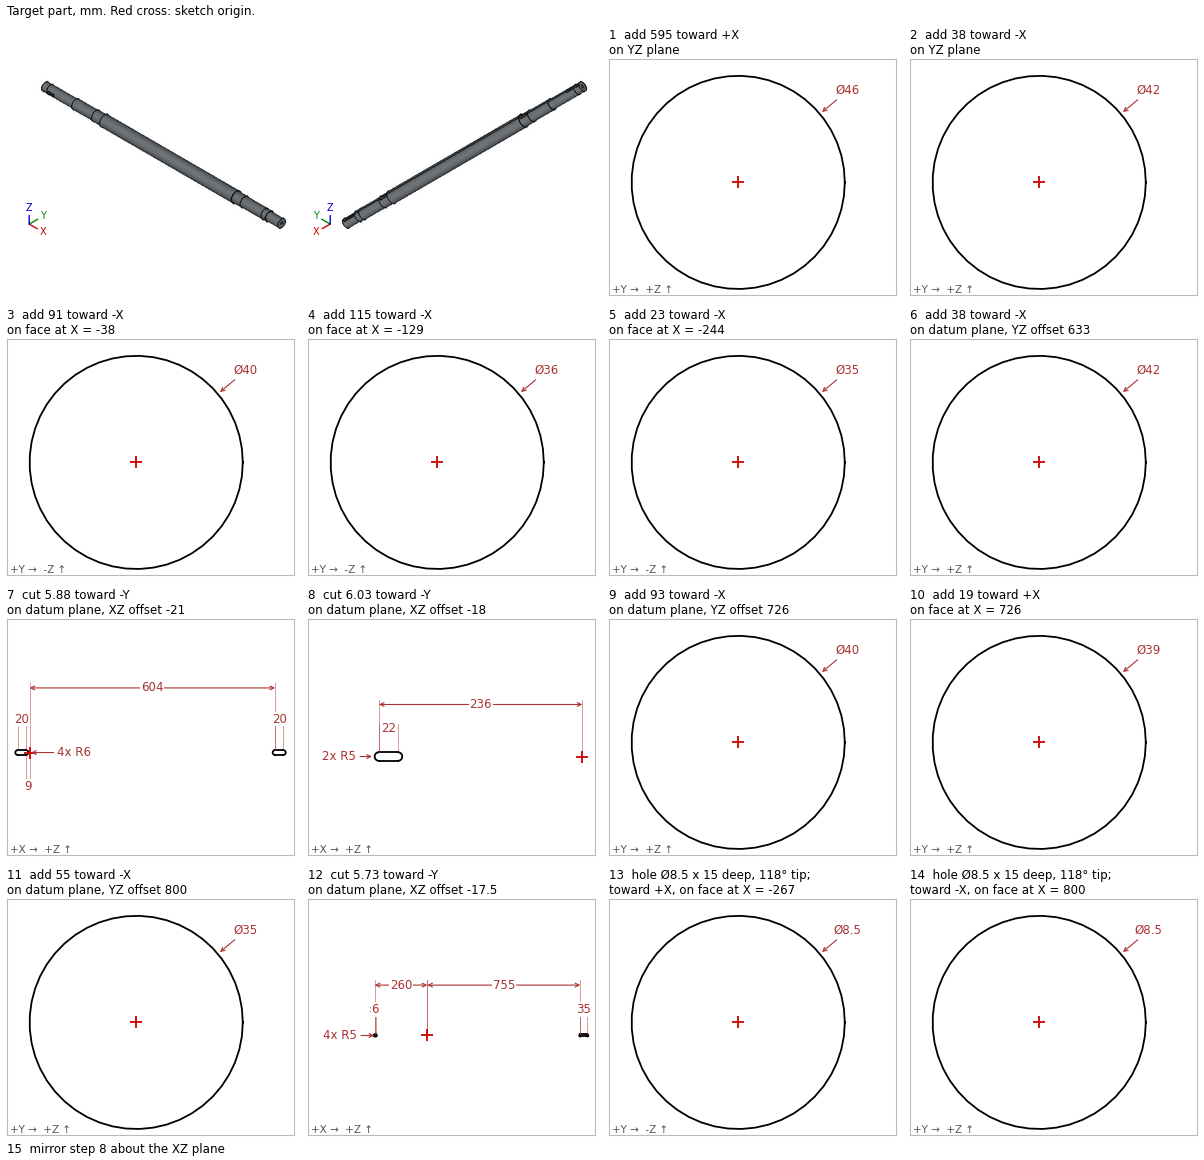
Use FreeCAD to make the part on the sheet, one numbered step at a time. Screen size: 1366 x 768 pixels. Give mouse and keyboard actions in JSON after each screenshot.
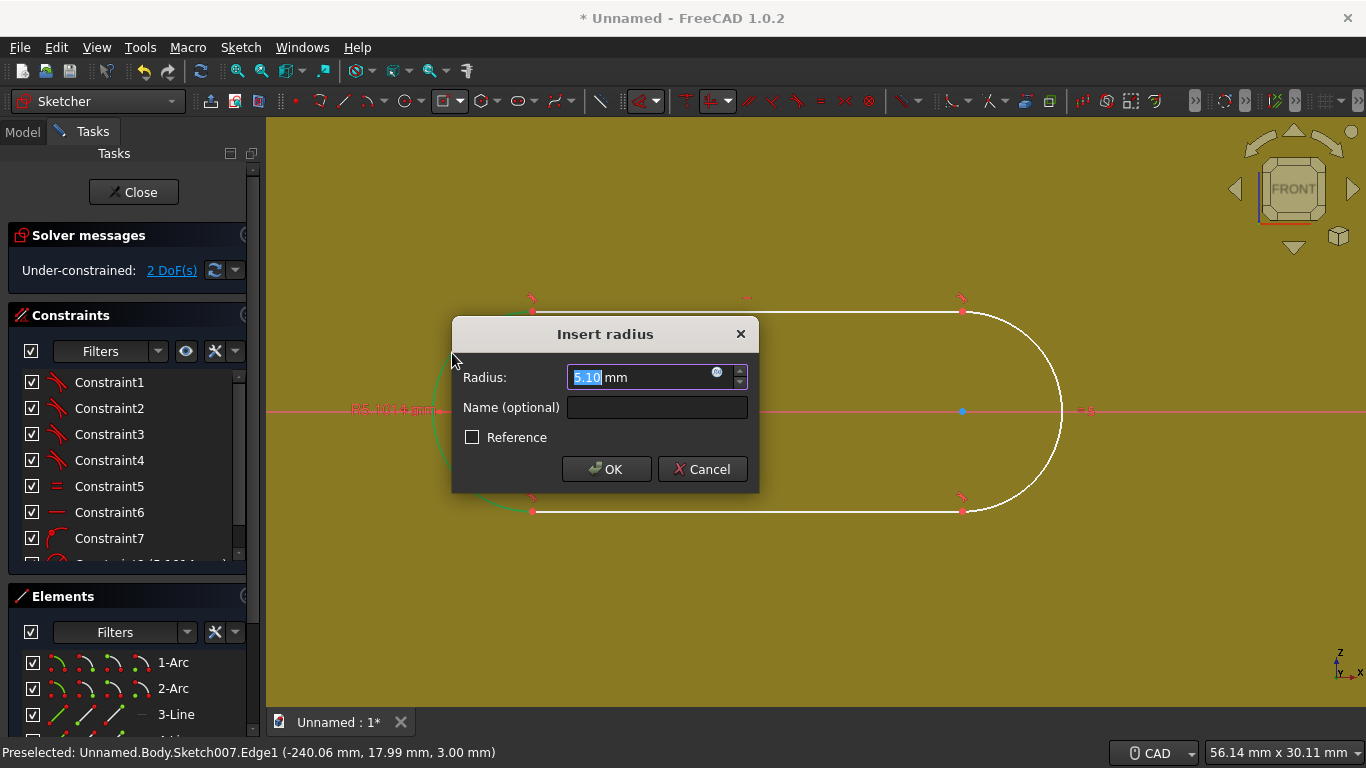
{"action": "type", "text": "5"}
{"action": "key", "text": "Return"}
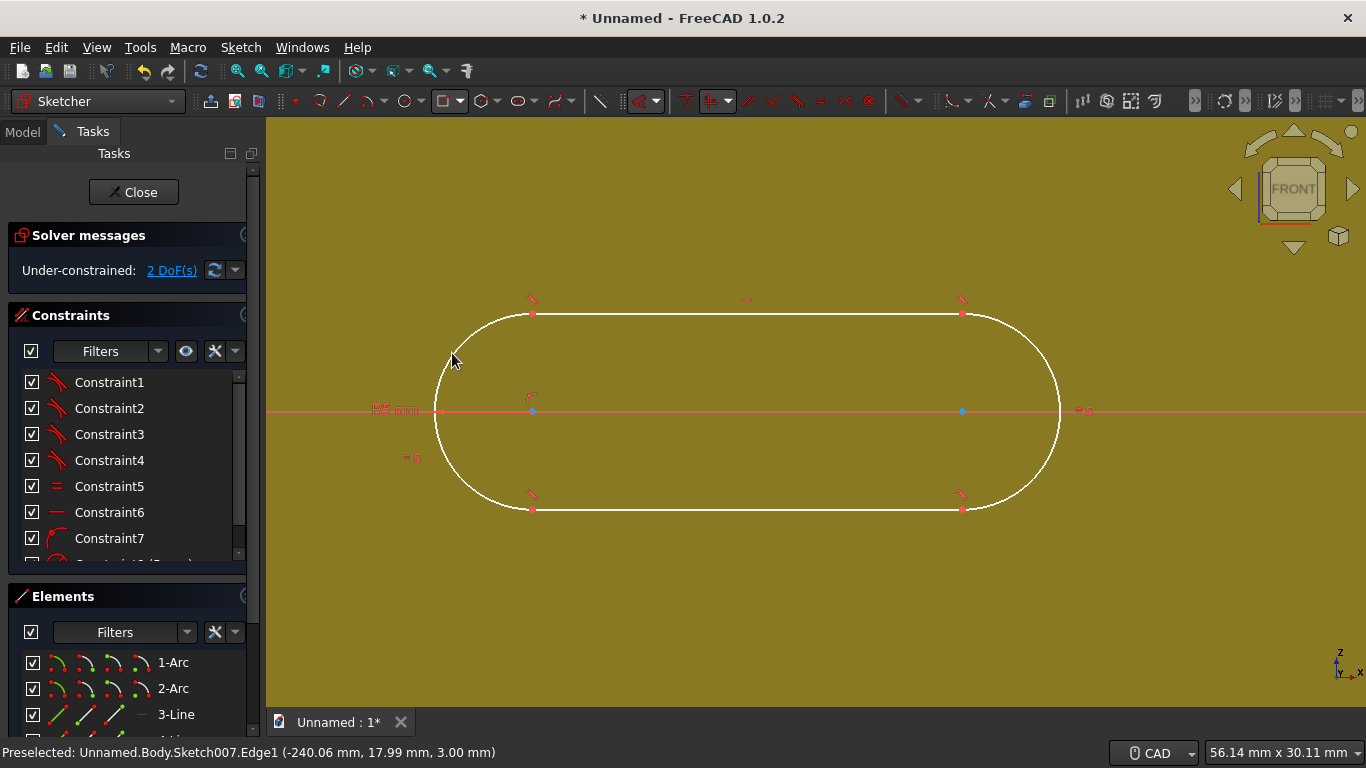
{"action": "left_click", "coordinate": [662, 314]}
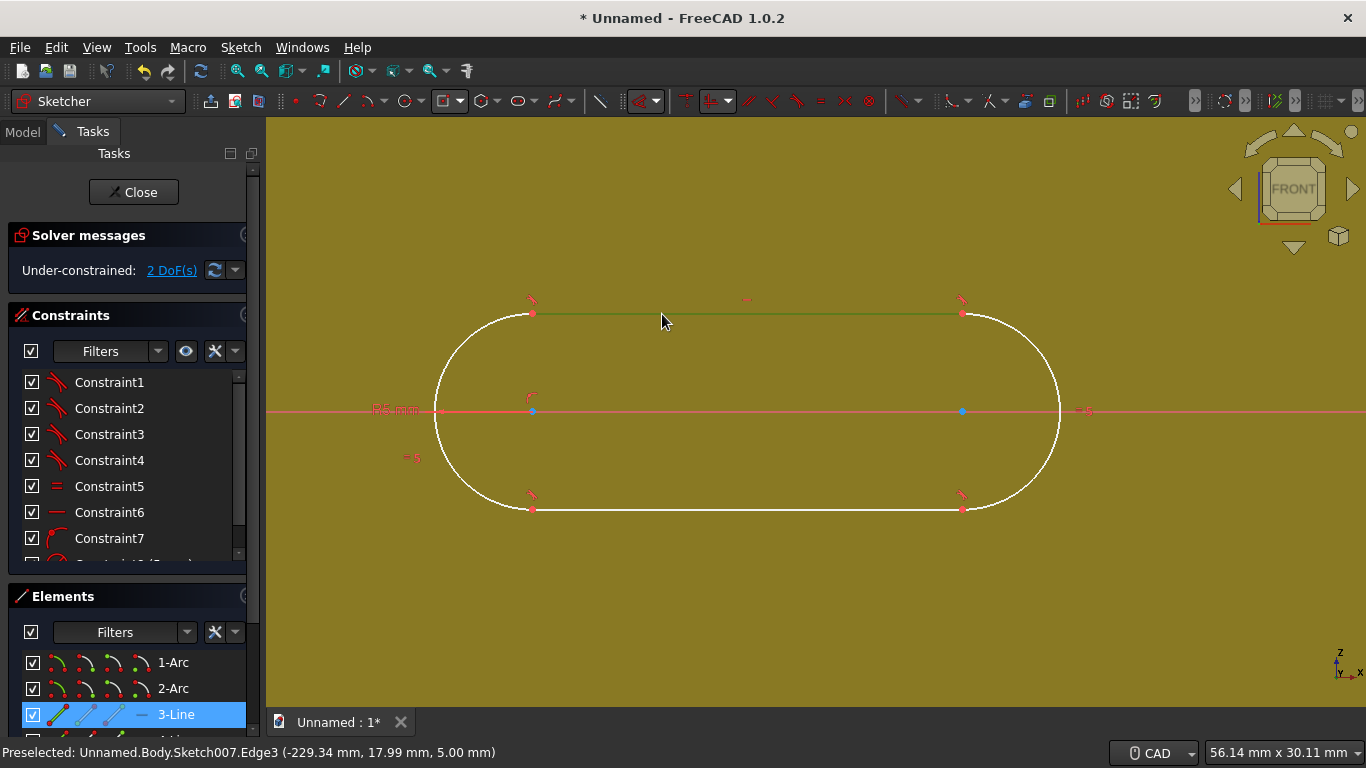
{"action": "key", "text": "l"}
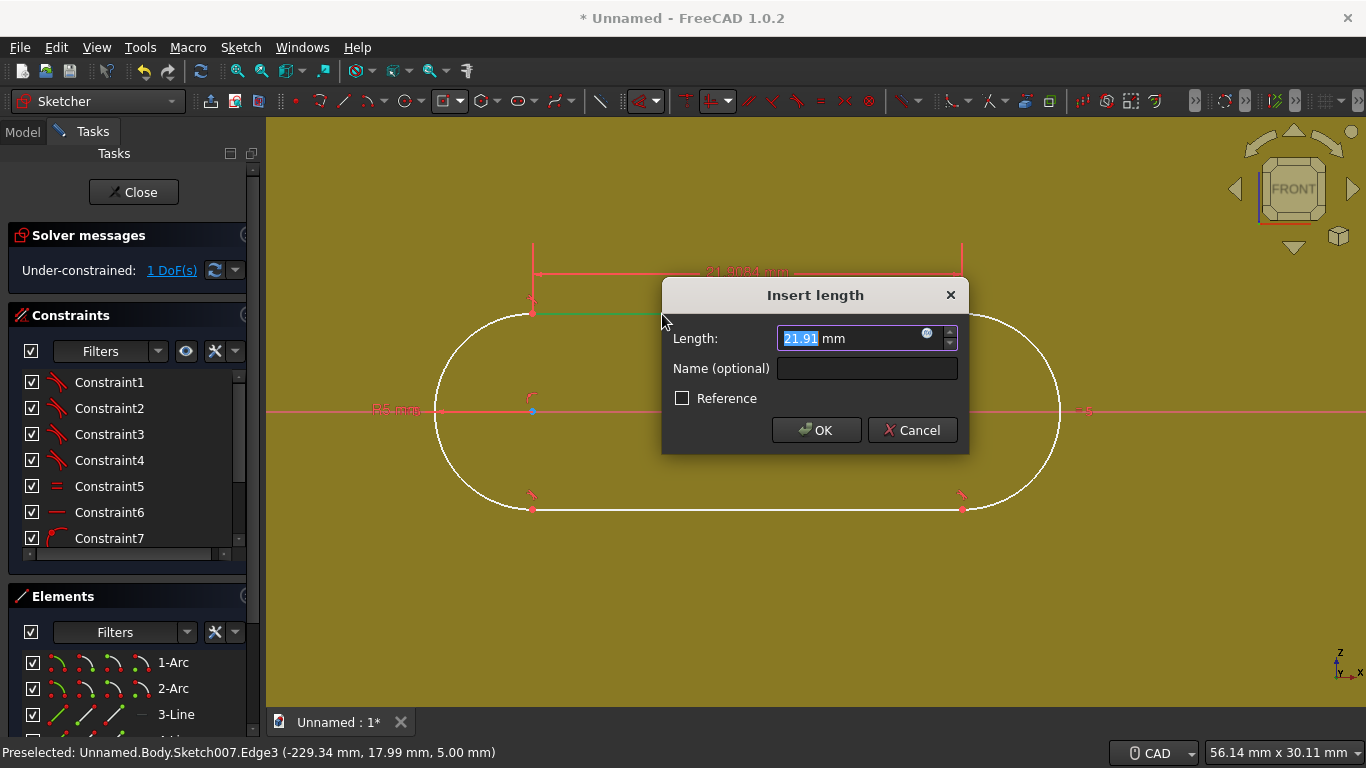
{"action": "type", "text": "22"}
{"action": "key", "text": "Return"}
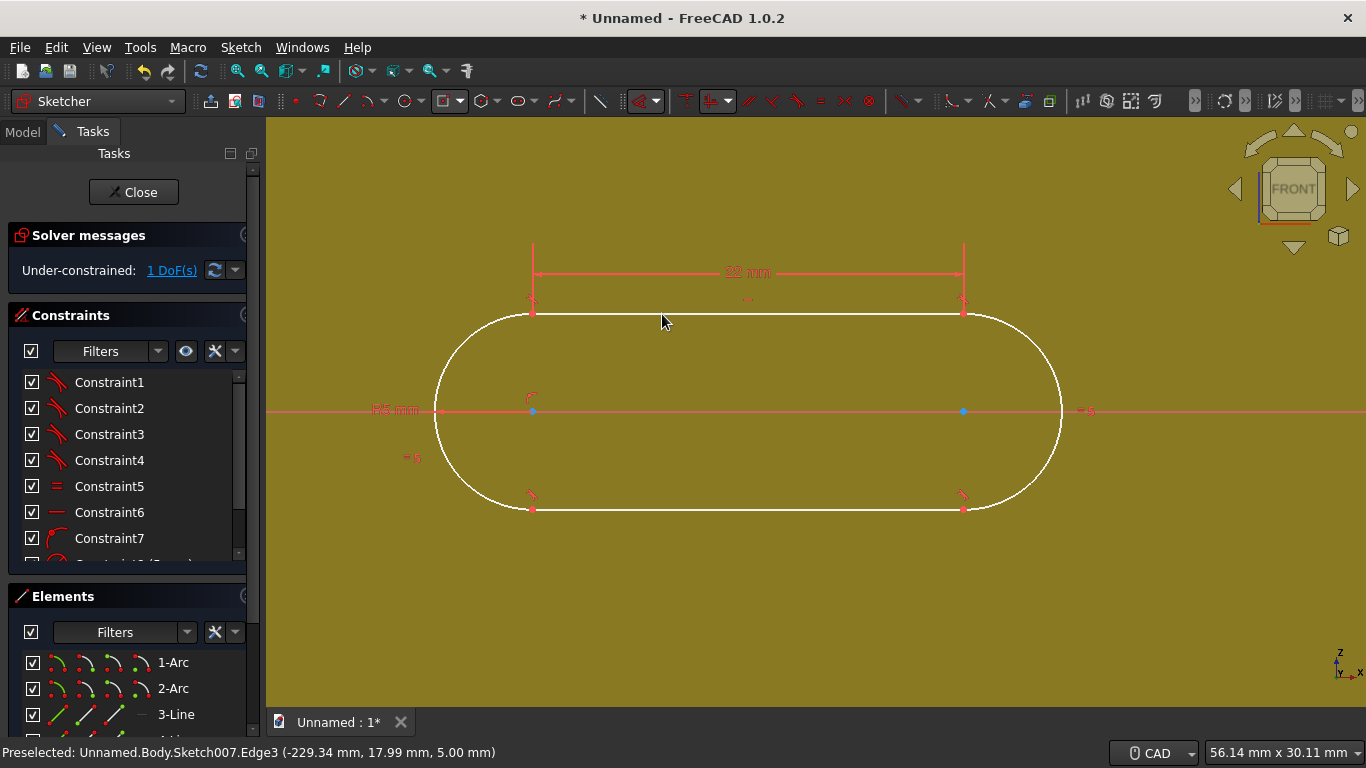
{"action": "left_click", "coordinate": [533, 314]}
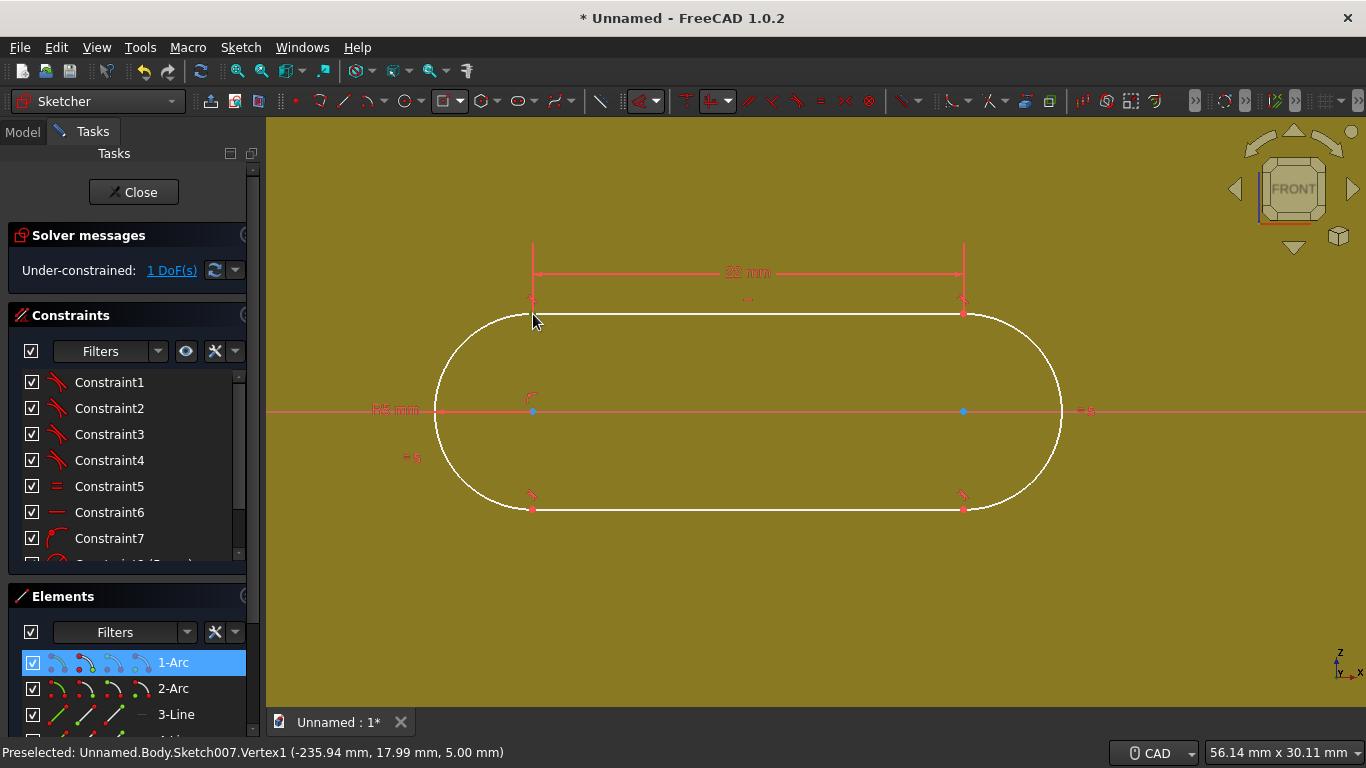
{"action": "key", "text": "l"}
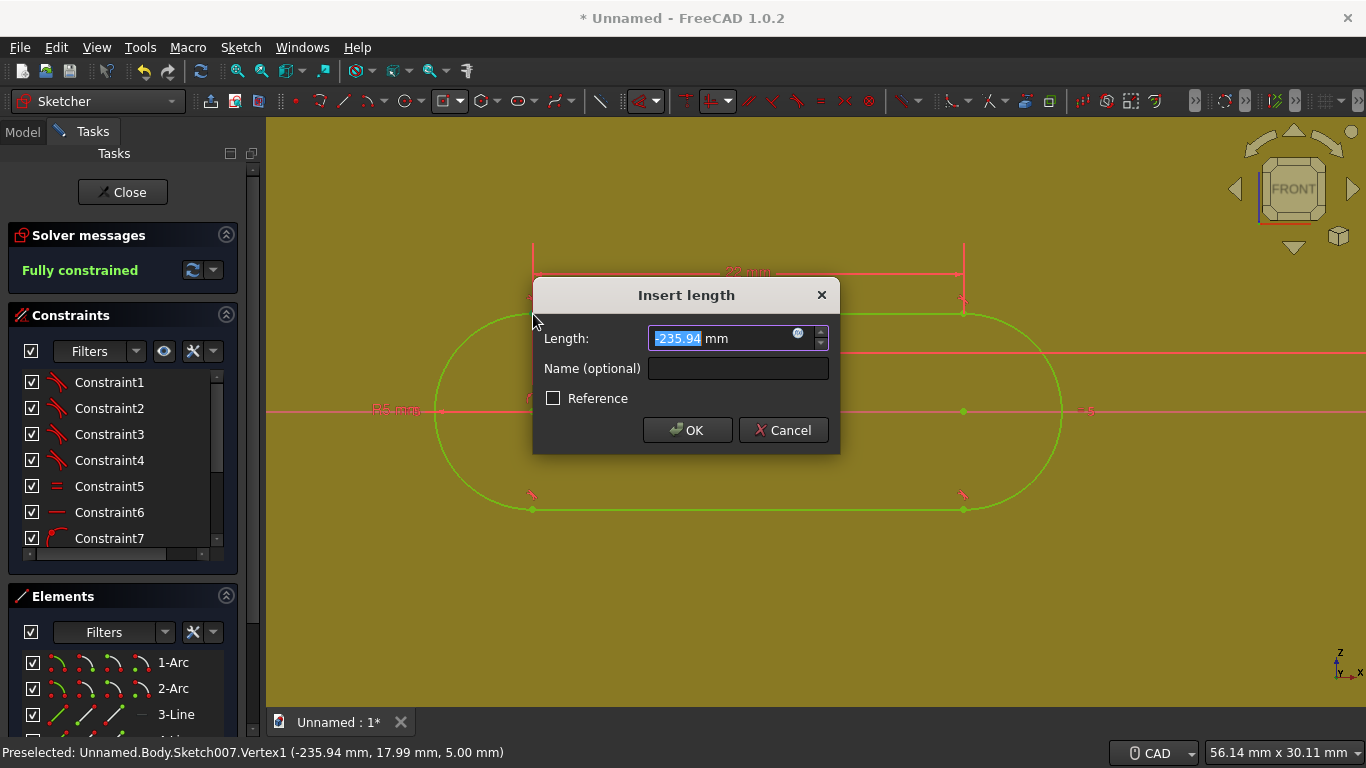
{"action": "type", "text": "-236"}
{"action": "key", "text": "Return"}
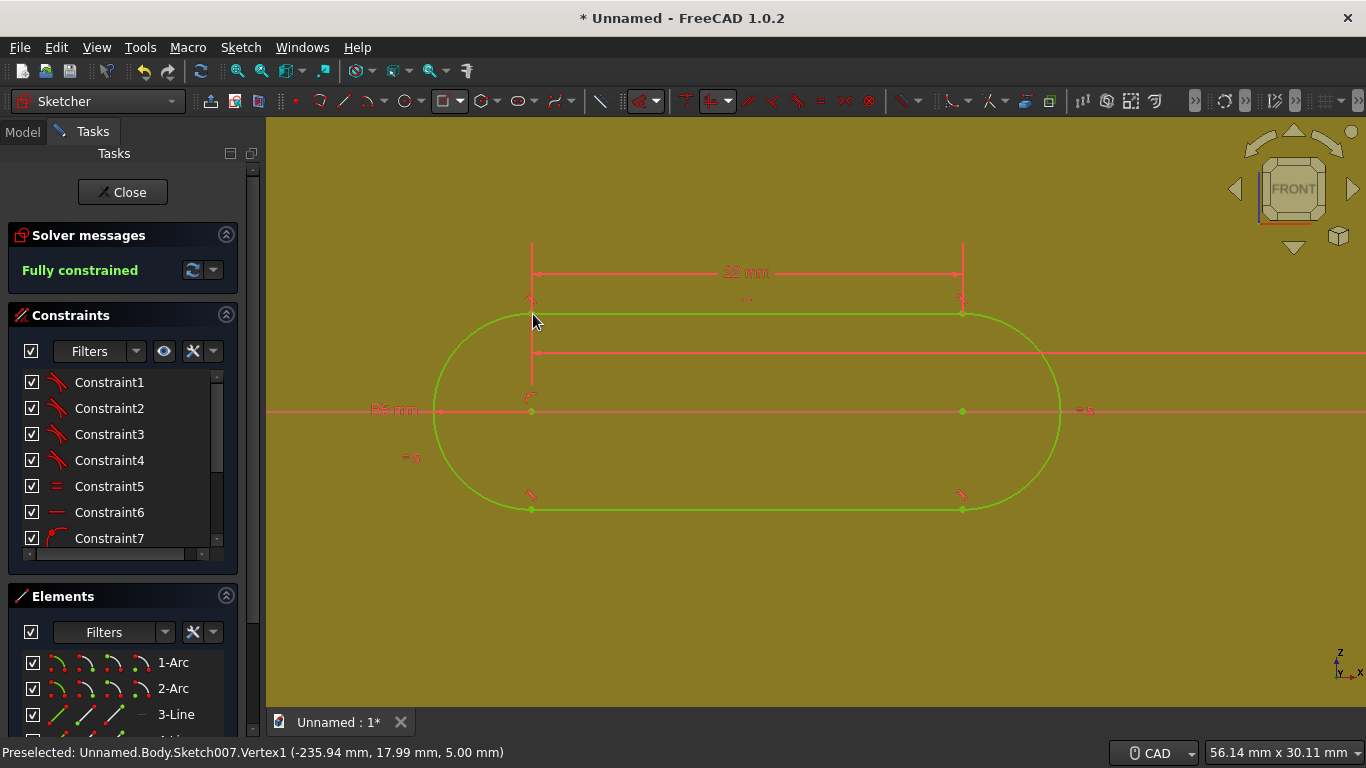
{"action": "left_click", "coordinate": [123, 192]}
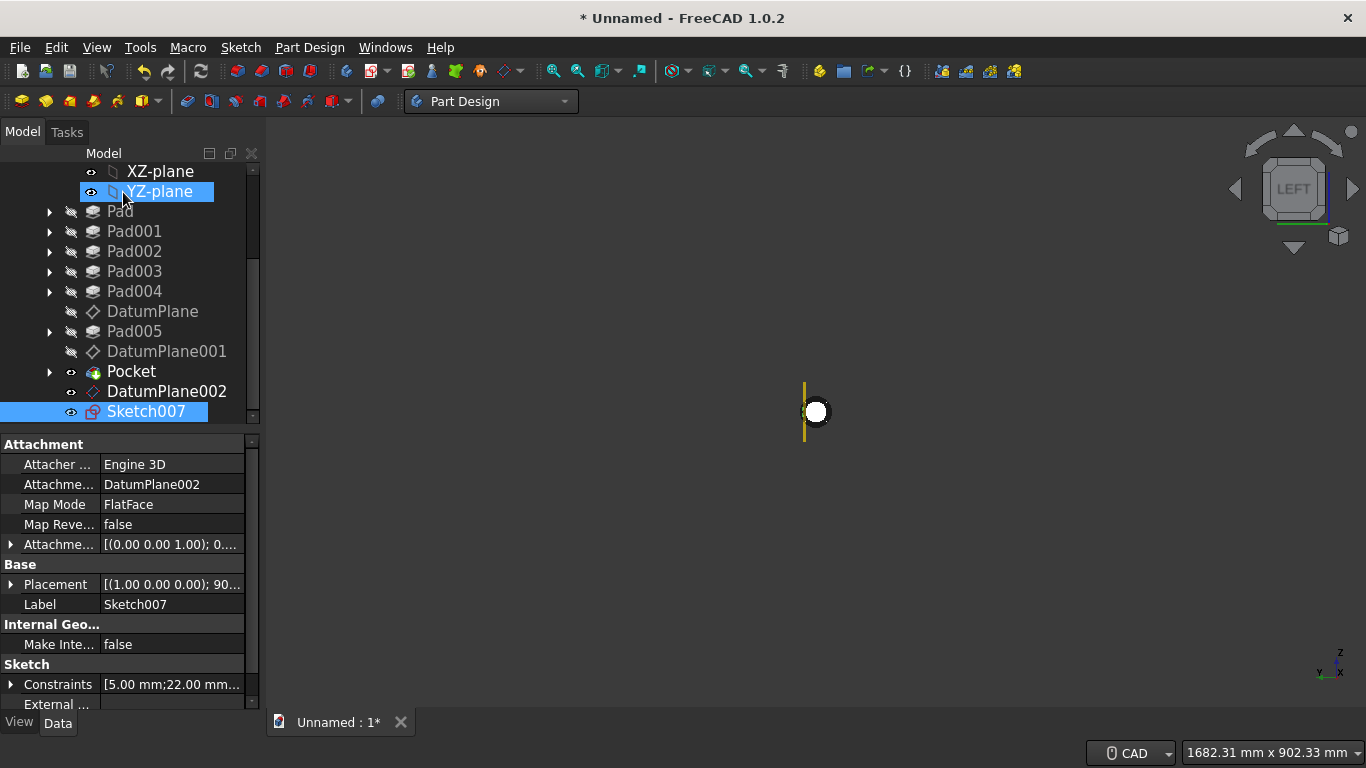
{"action": "left_click", "coordinate": [188, 102]}